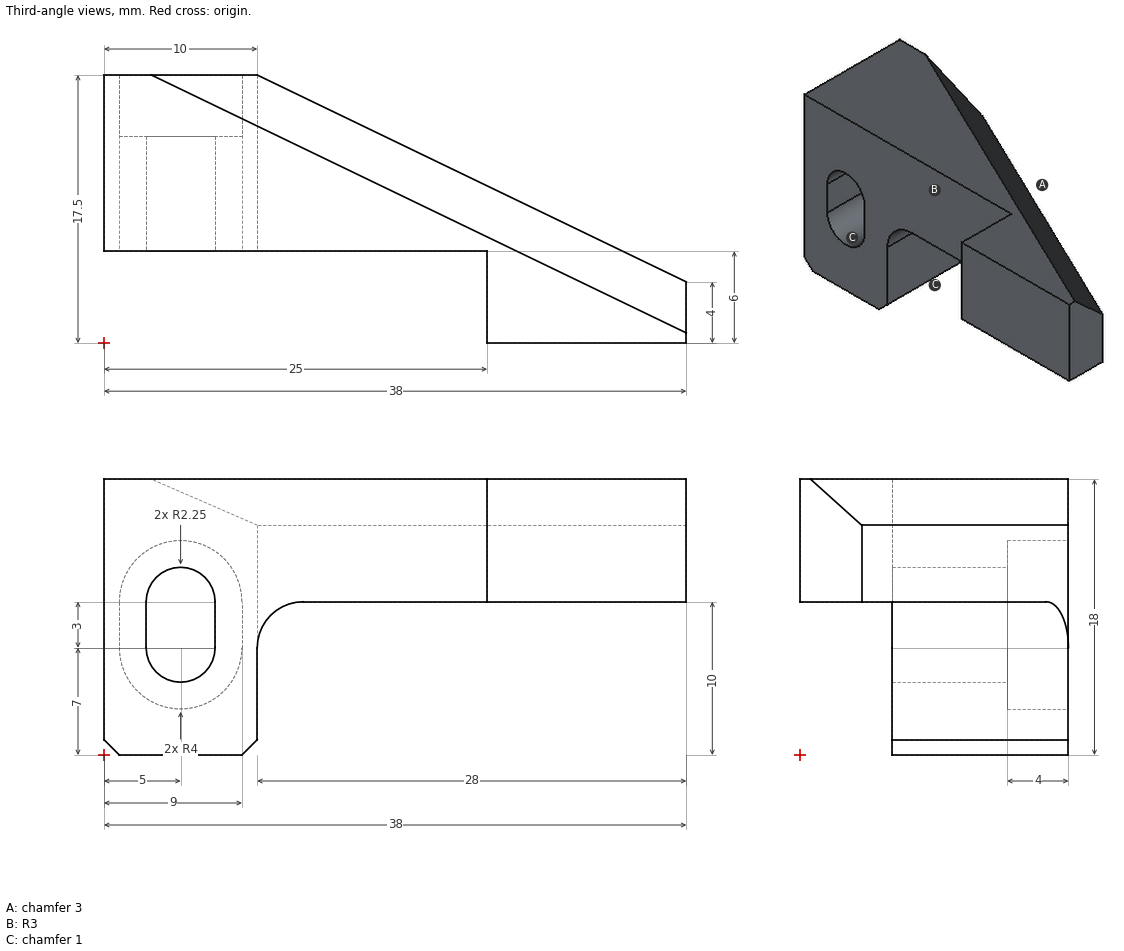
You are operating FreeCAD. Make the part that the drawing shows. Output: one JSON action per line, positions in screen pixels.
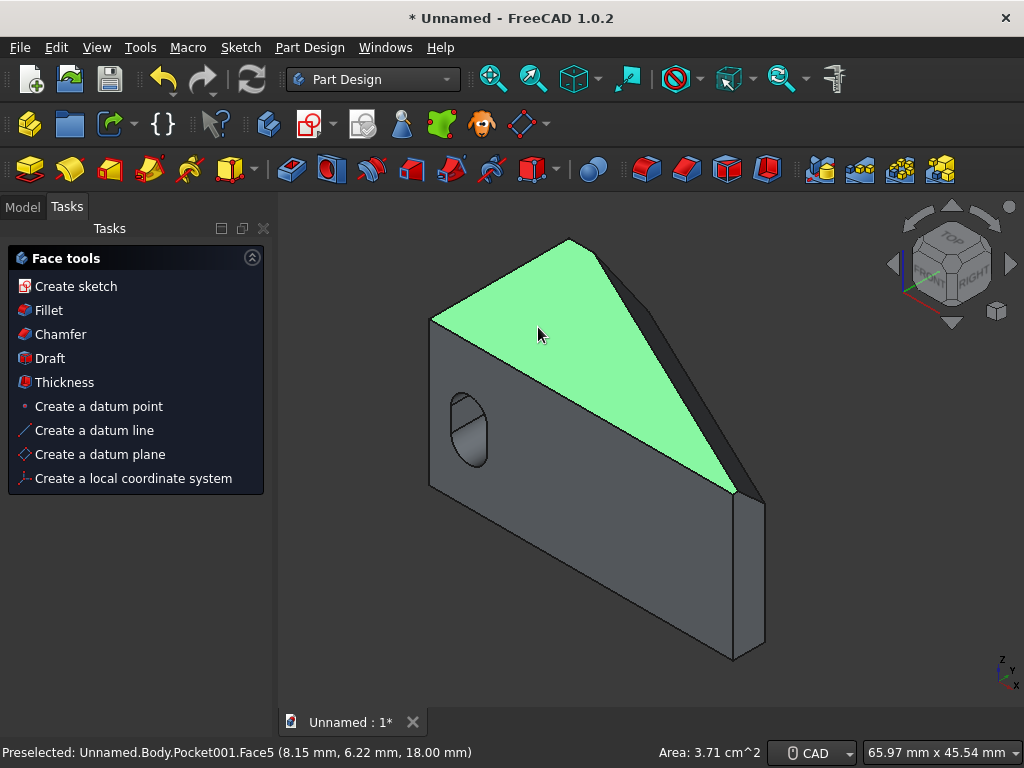
{"action": "left_click", "coordinate": [310, 124]}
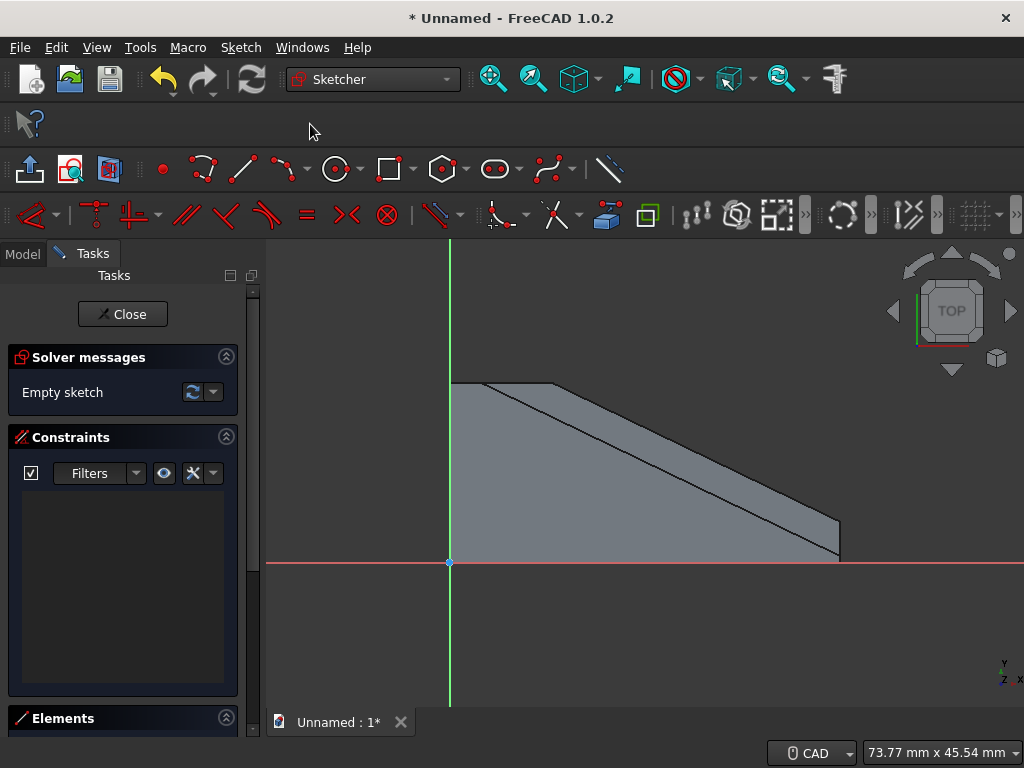
{"action": "scroll", "coordinate": [582, 652], "scroll_direction": "up", "scroll_amount": 2}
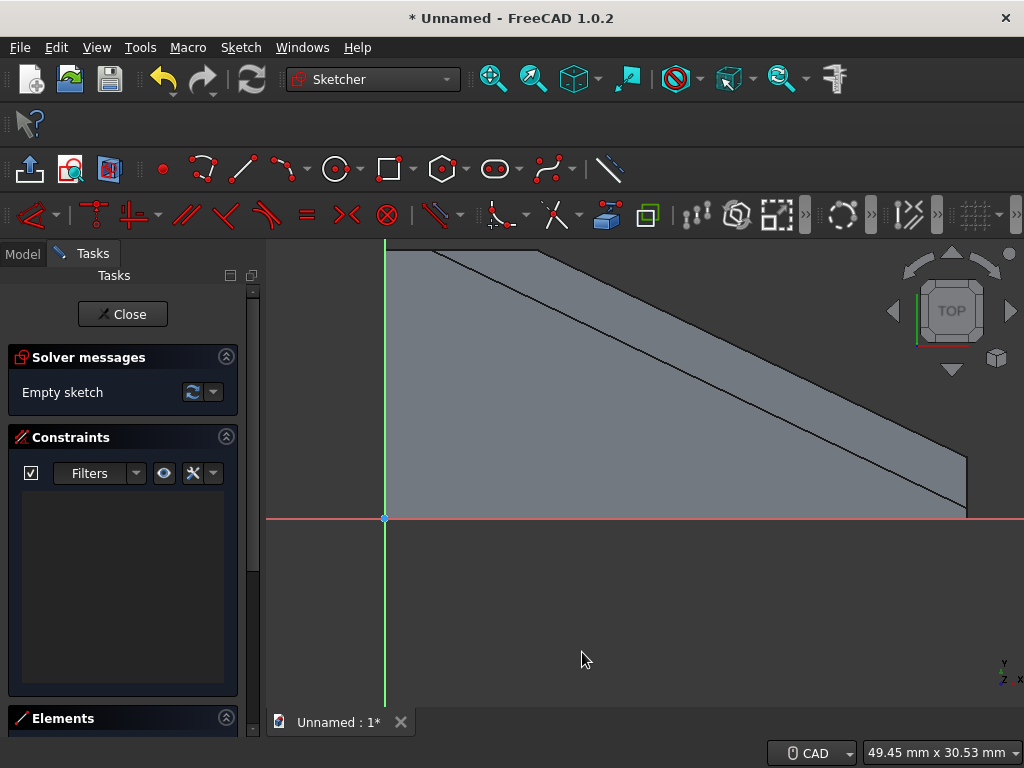
{"action": "key", "text": "g r"}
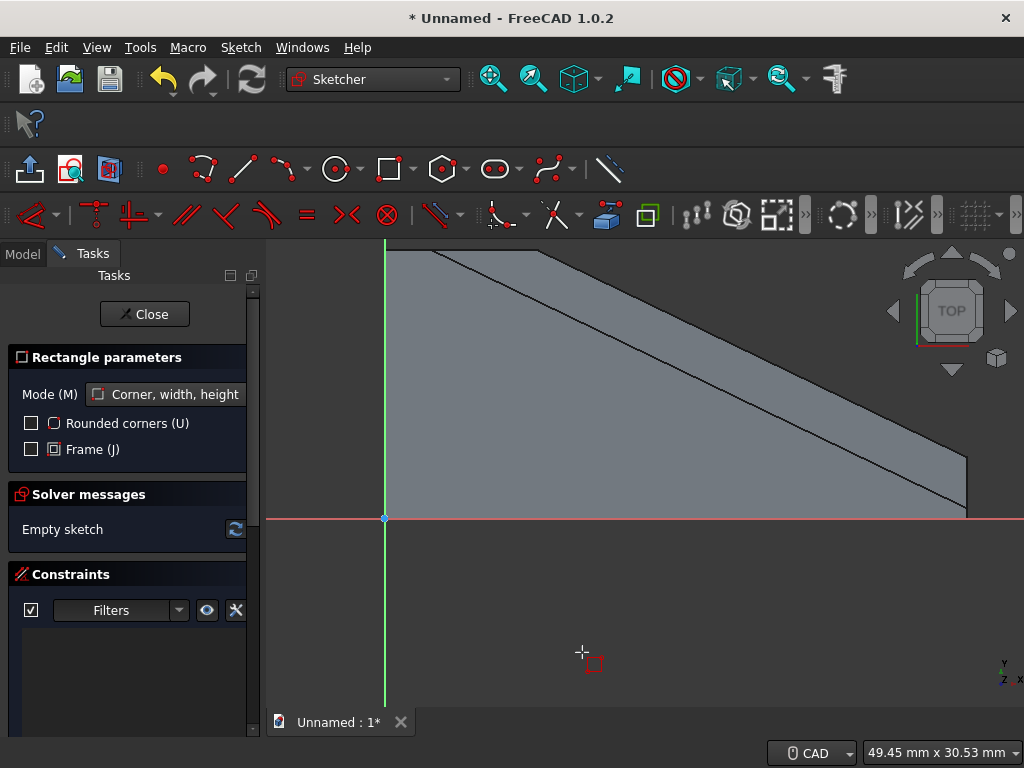
{"action": "left_click", "coordinate": [385, 519]}
{"action": "mouse_move", "coordinate": [768, 427]}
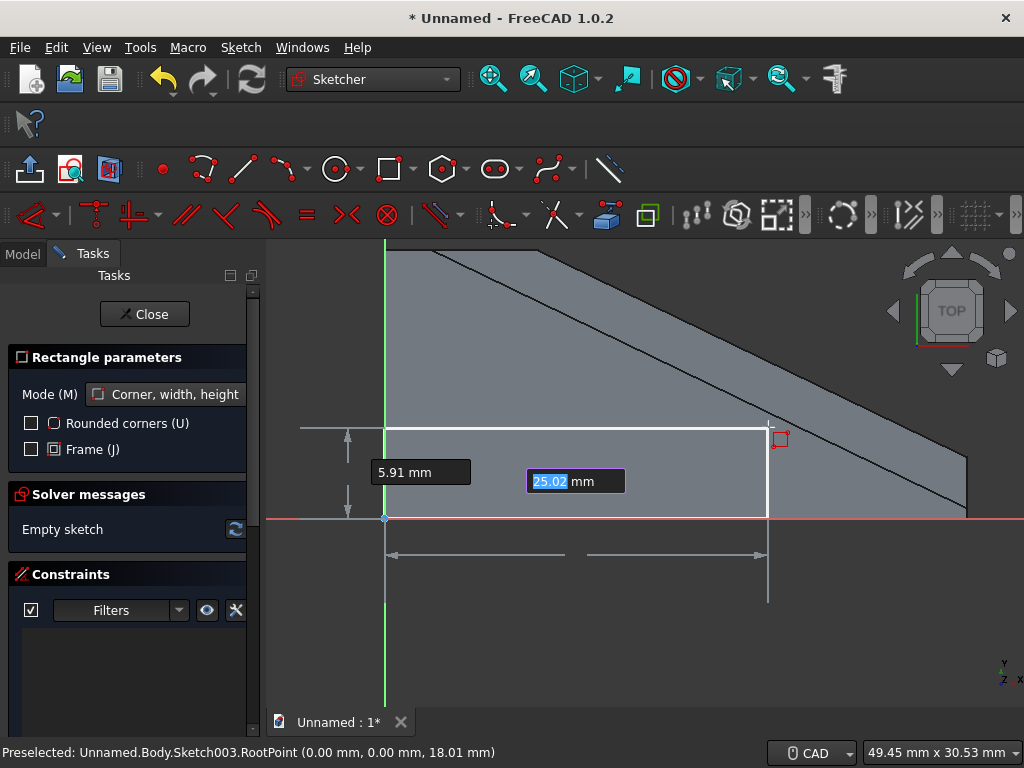
{"action": "type", "text": "25"}
{"action": "key", "text": "Tab"}
{"action": "type", "text": "6"}
{"action": "key", "text": "Return"}
{"action": "key", "text": "Escape"}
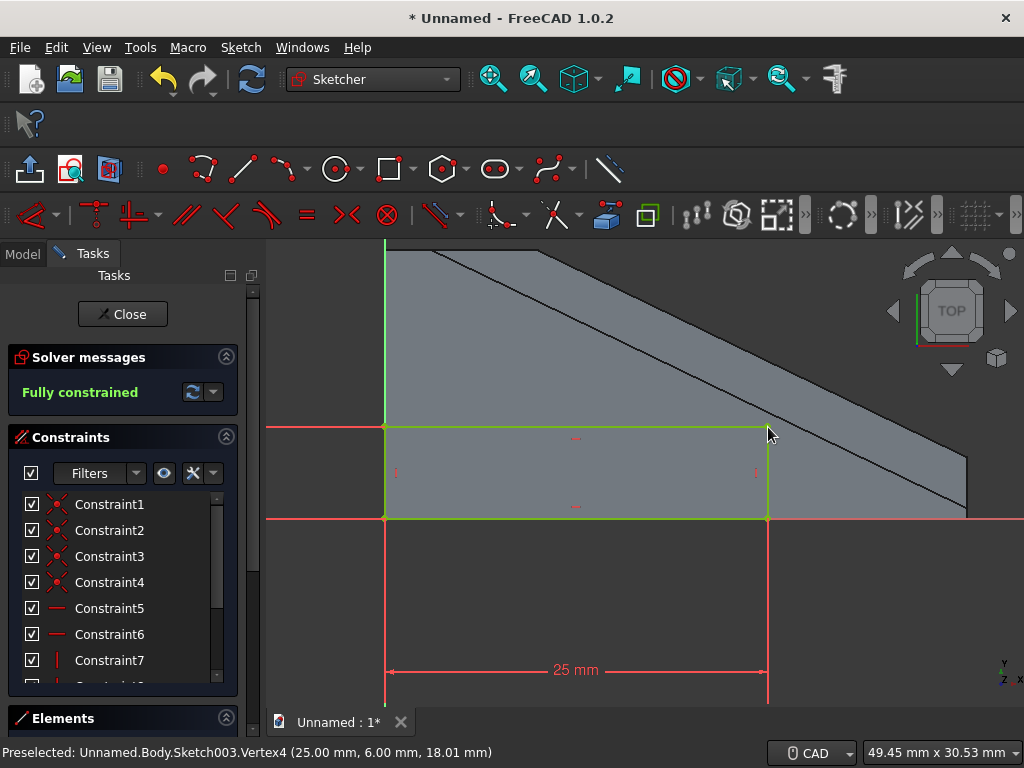
{"action": "left_click", "coordinate": [123, 314]}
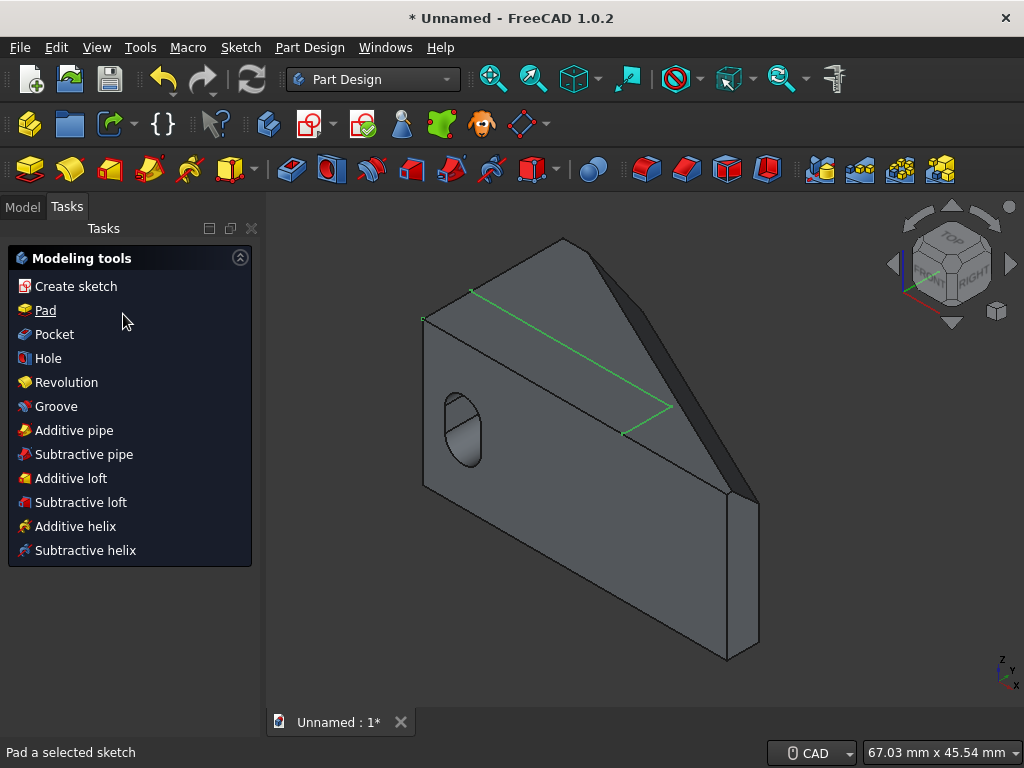
{"action": "left_click", "coordinate": [292, 170]}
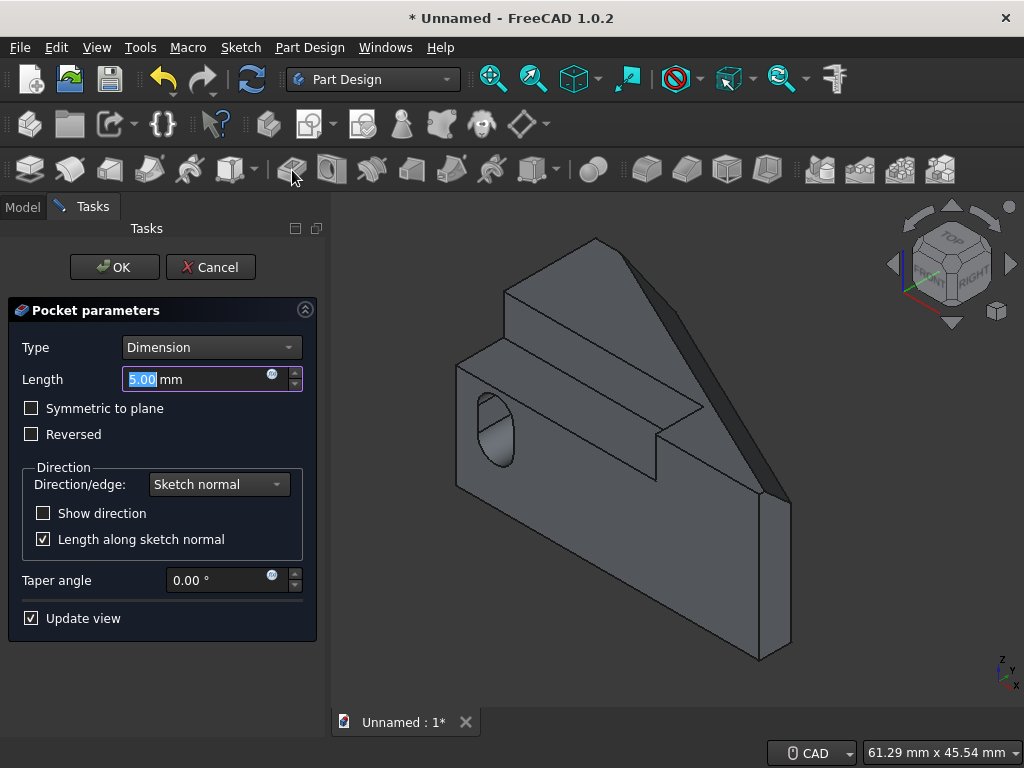
{"action": "left_click", "coordinate": [212, 348]}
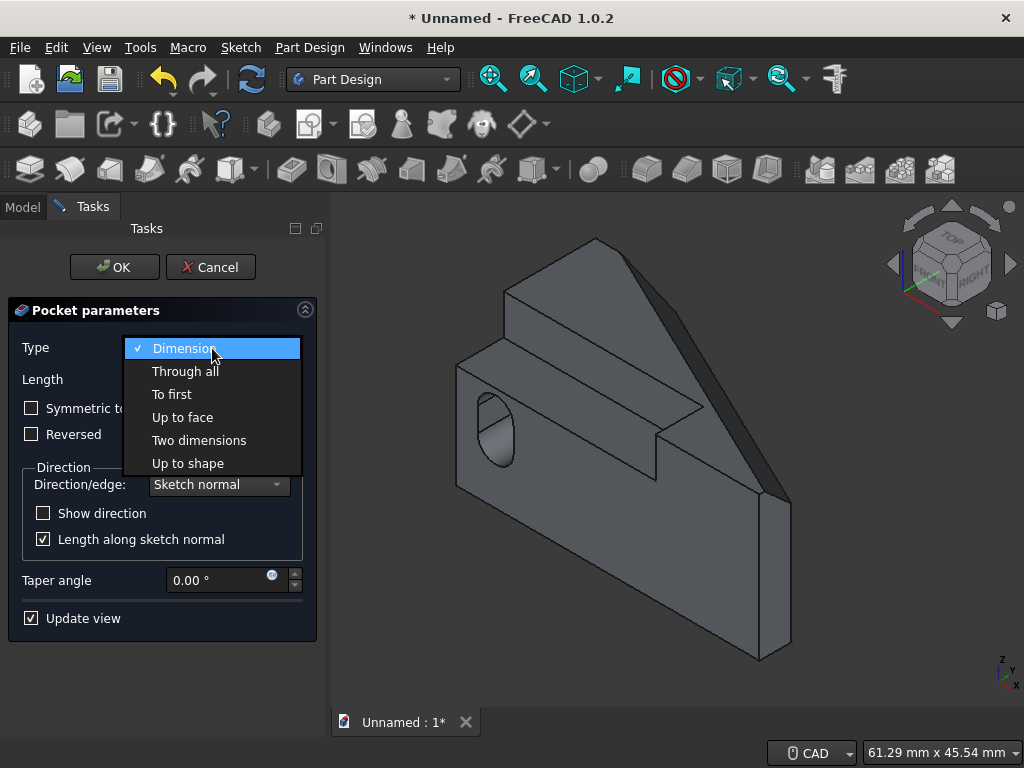
{"action": "left_click", "coordinate": [212, 372]}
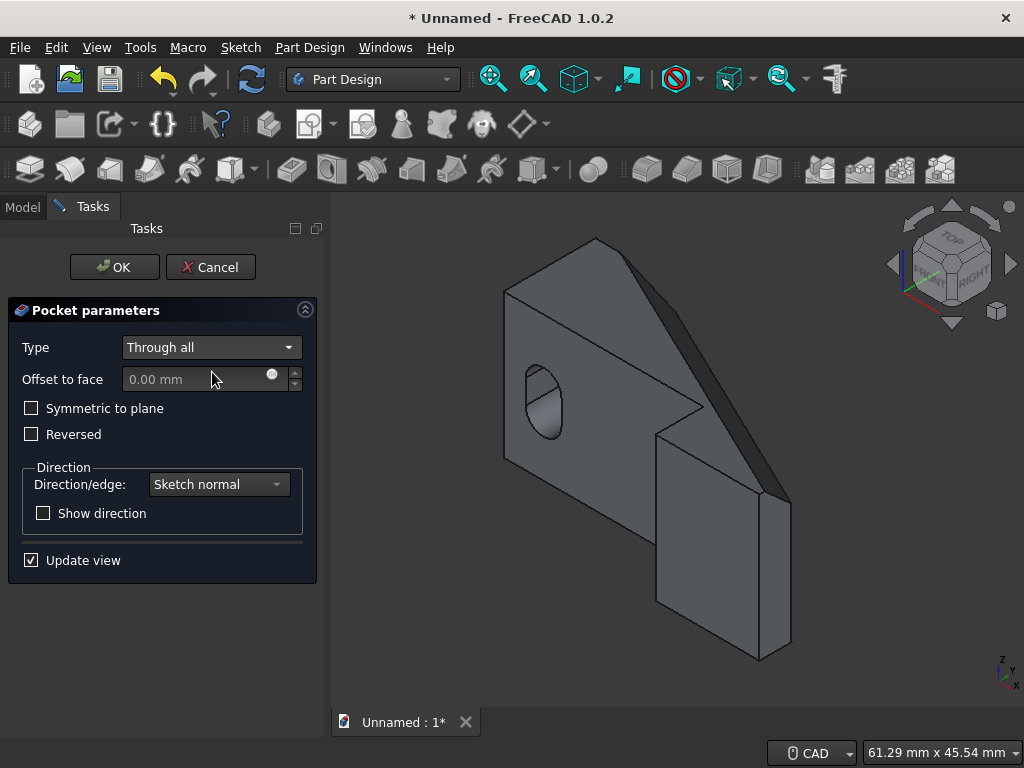
{"action": "left_click", "coordinate": [115, 267]}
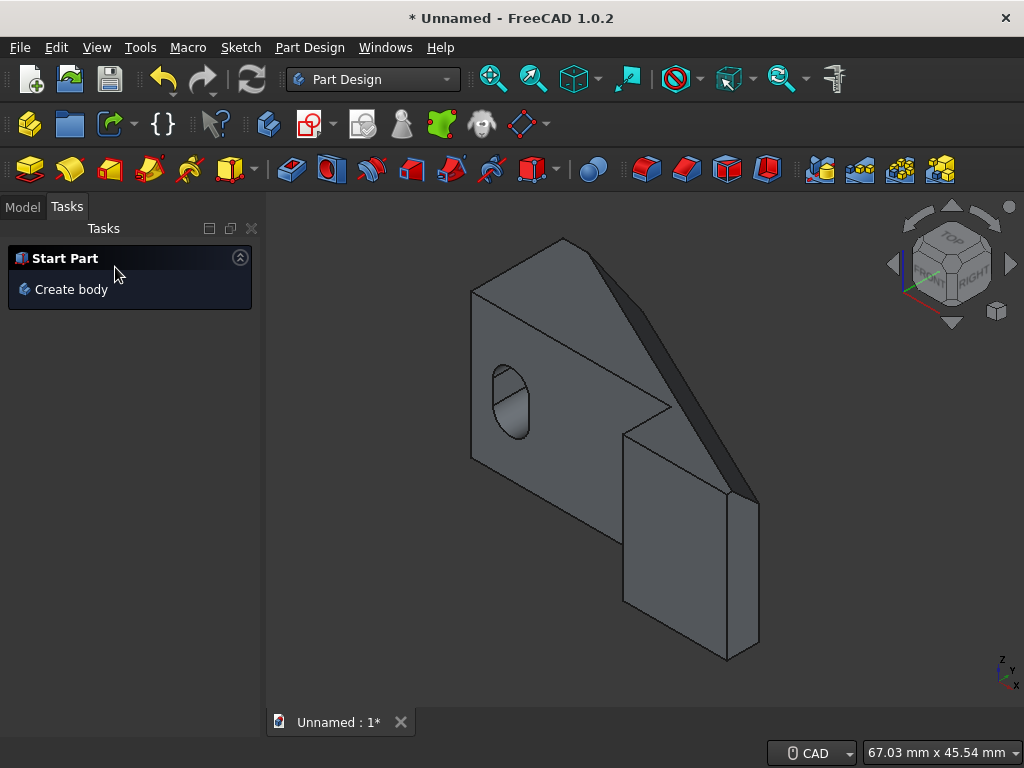
{"action": "key", "text": "4"}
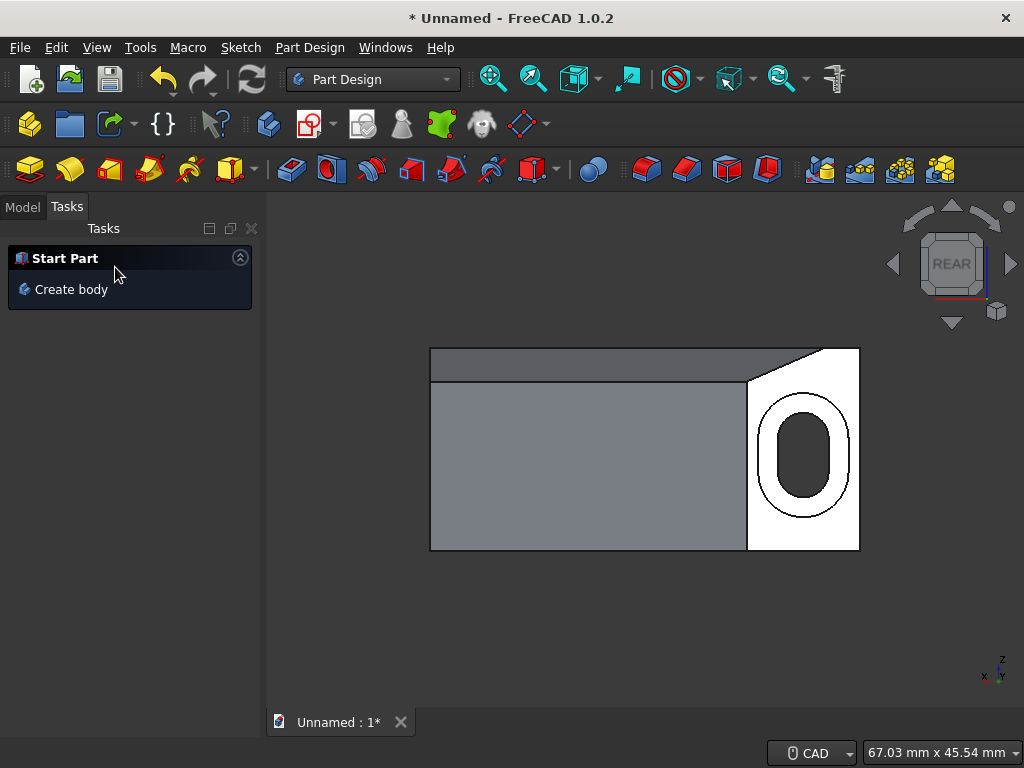
{"action": "left_click", "coordinate": [771, 536]}